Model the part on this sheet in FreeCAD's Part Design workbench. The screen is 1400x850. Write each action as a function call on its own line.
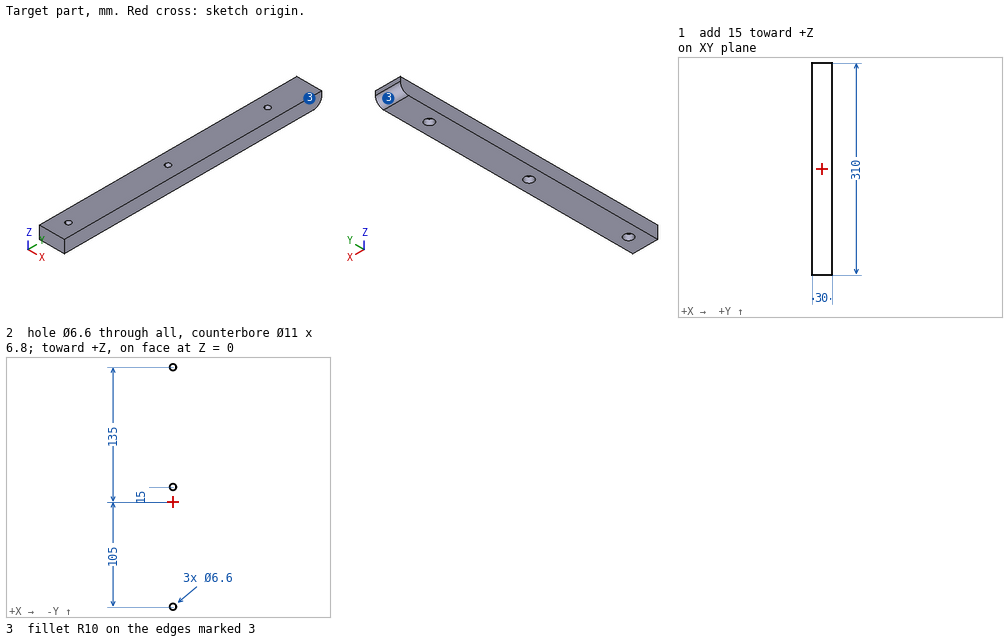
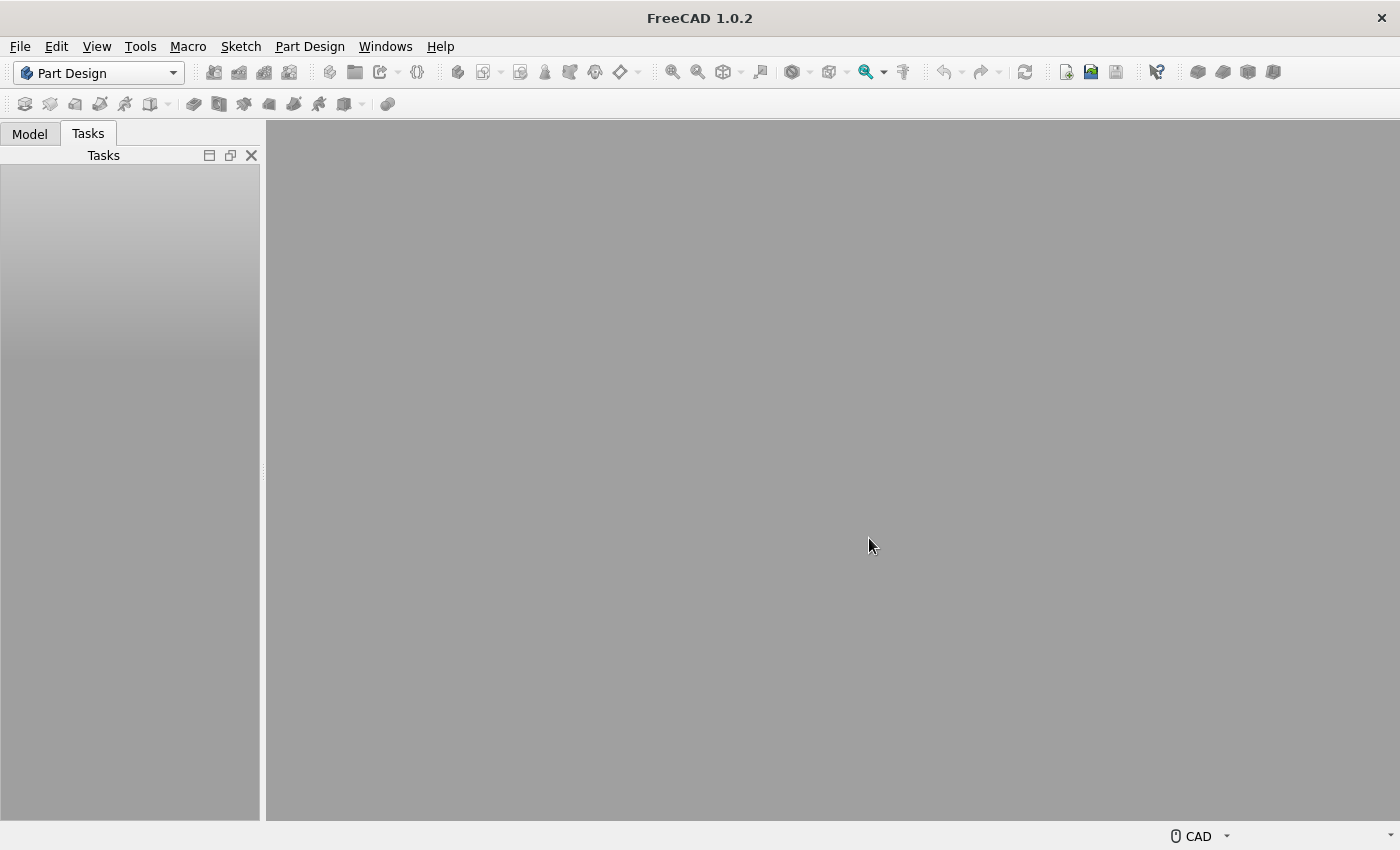
click(1066, 72)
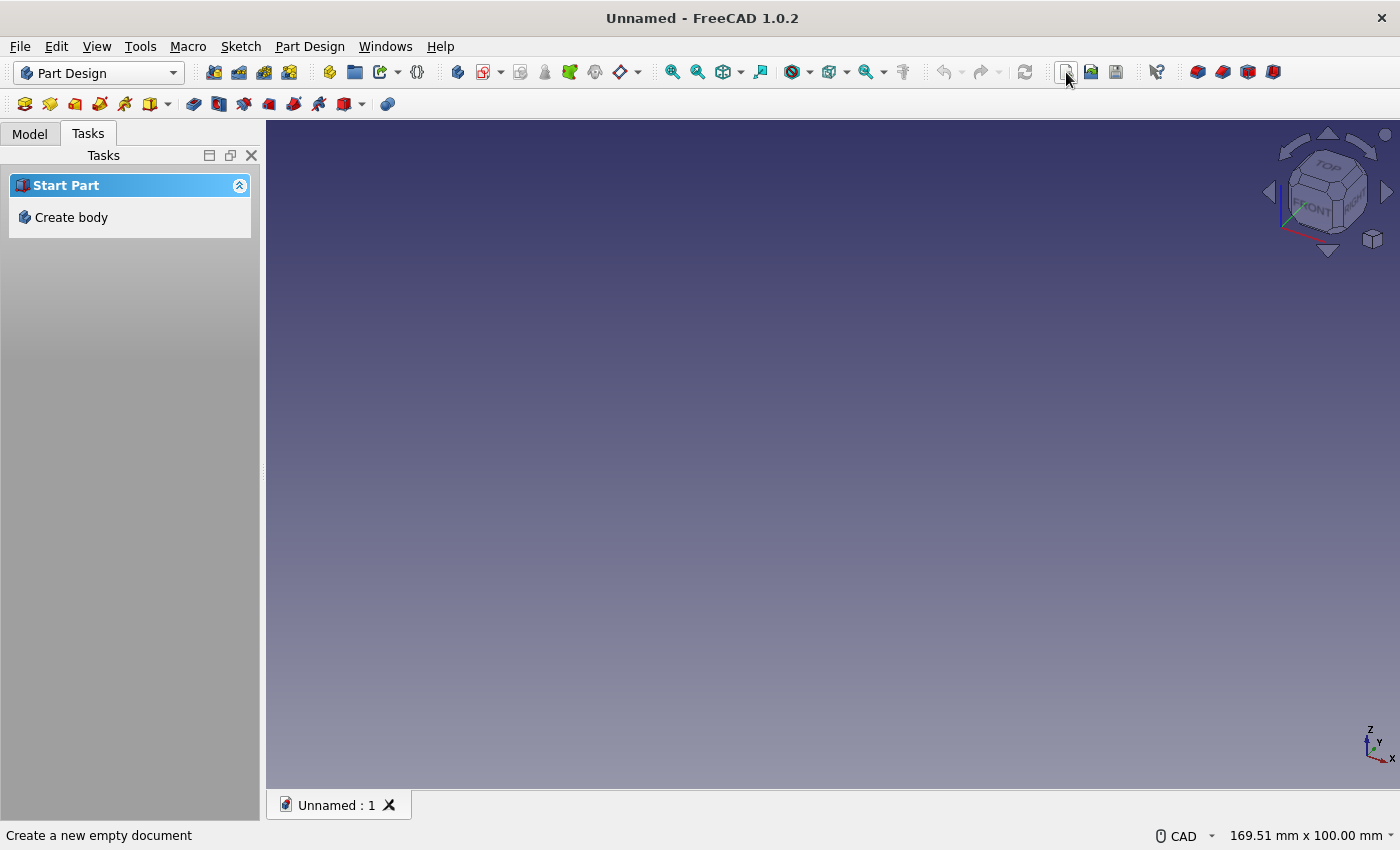
click(482, 72)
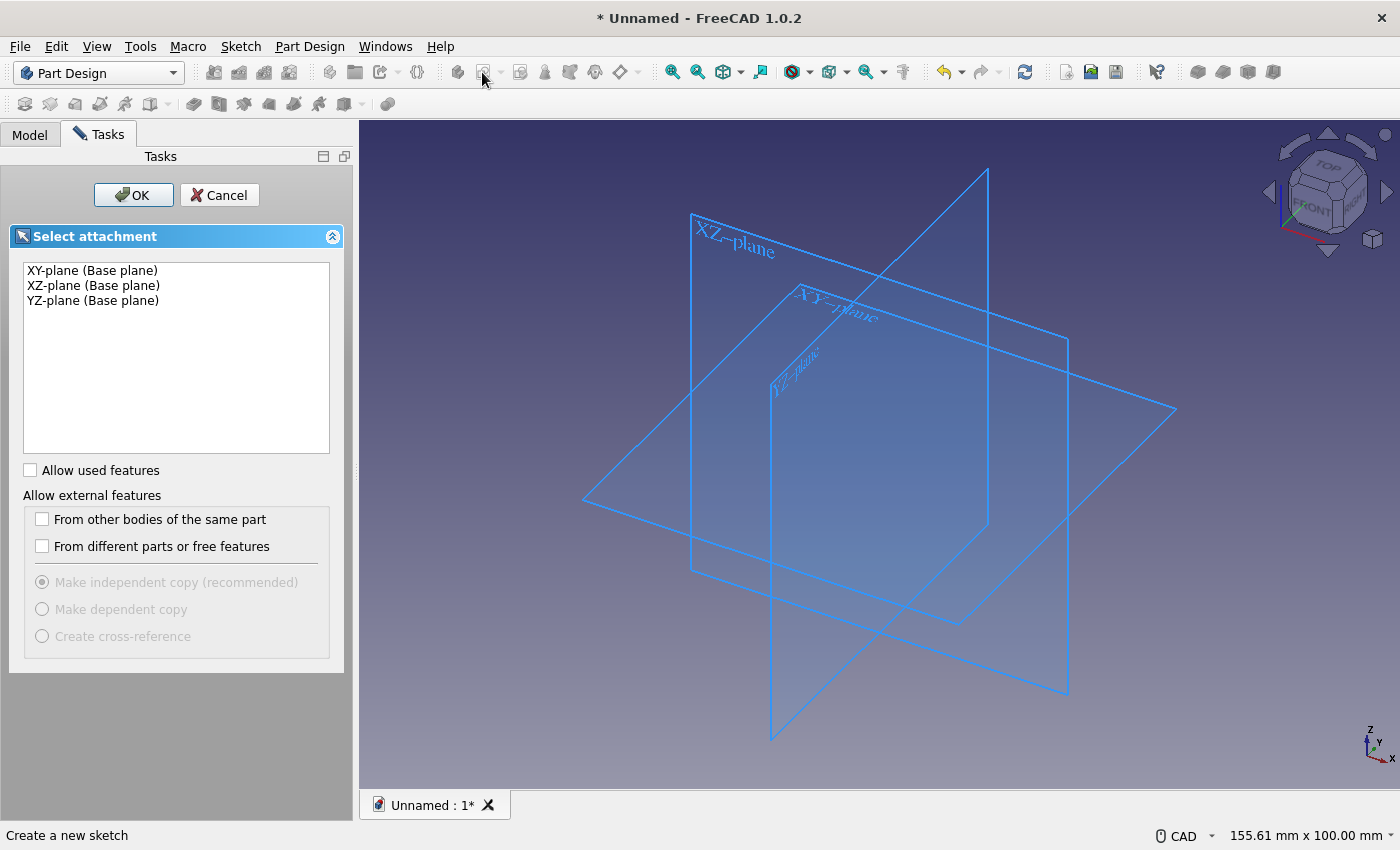
click(84, 270)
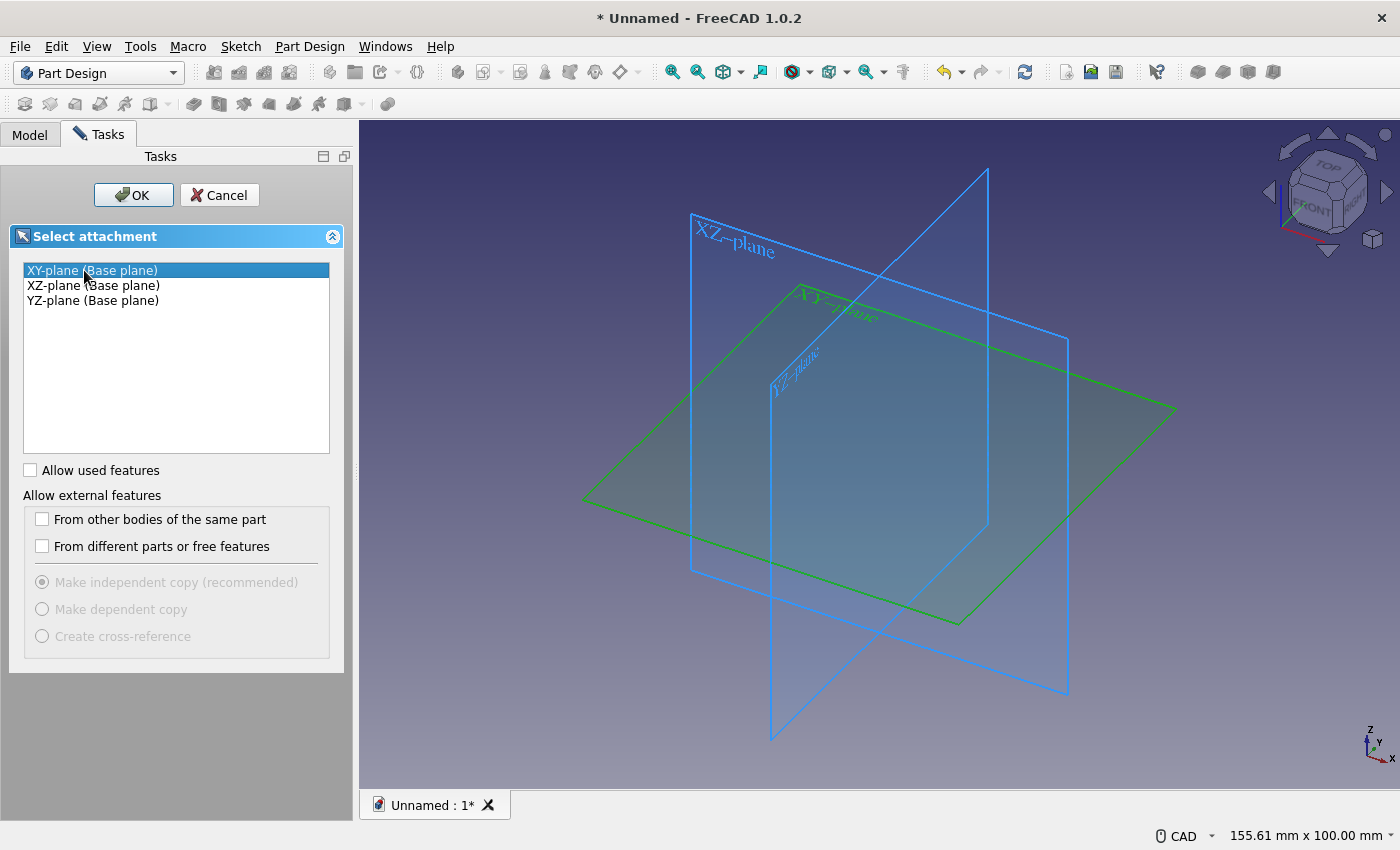
click(134, 195)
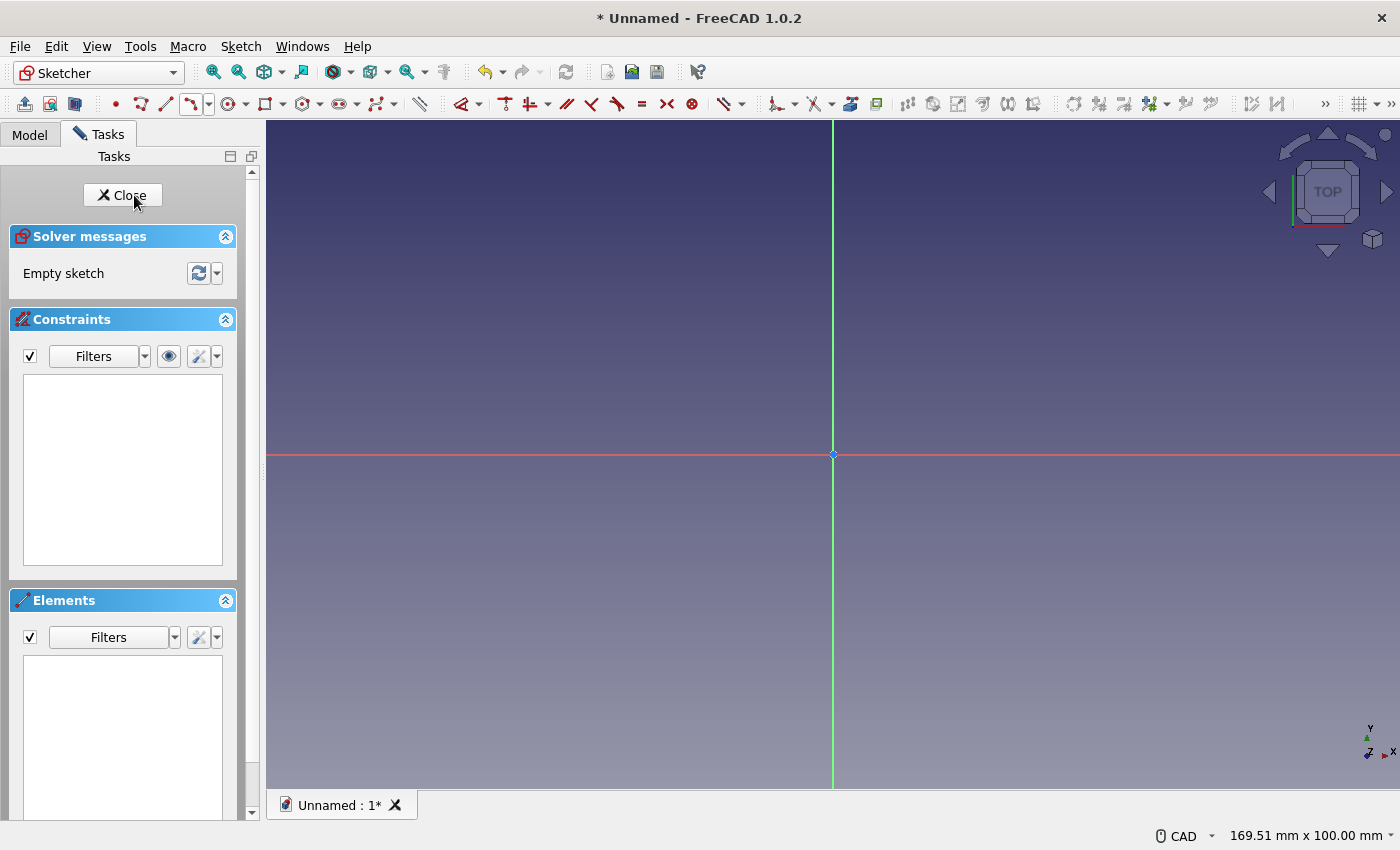
scroll(747, 454, down, 8)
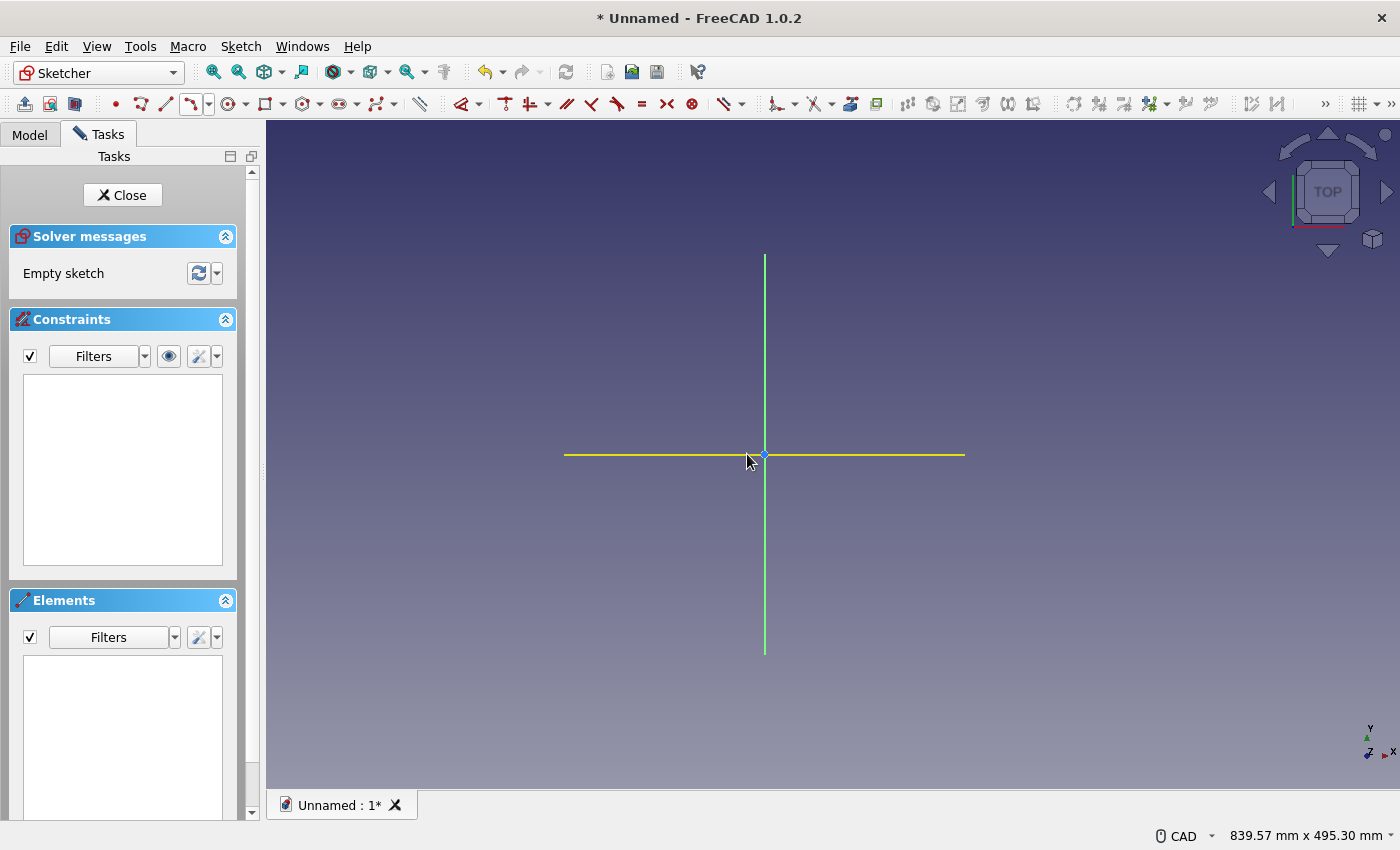
key(g)
key(v)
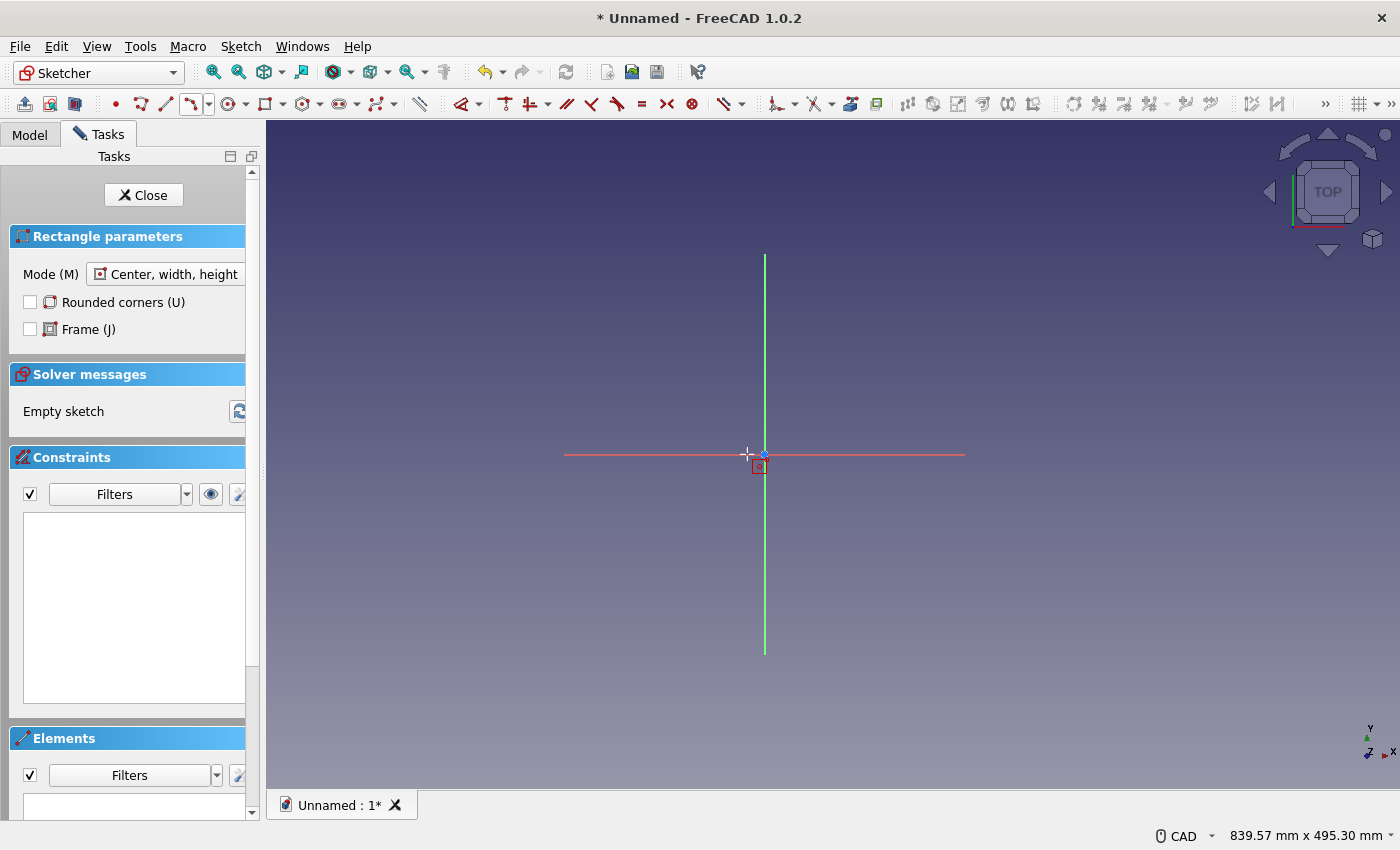
click(765, 454)
click(785, 245)
key(Escape)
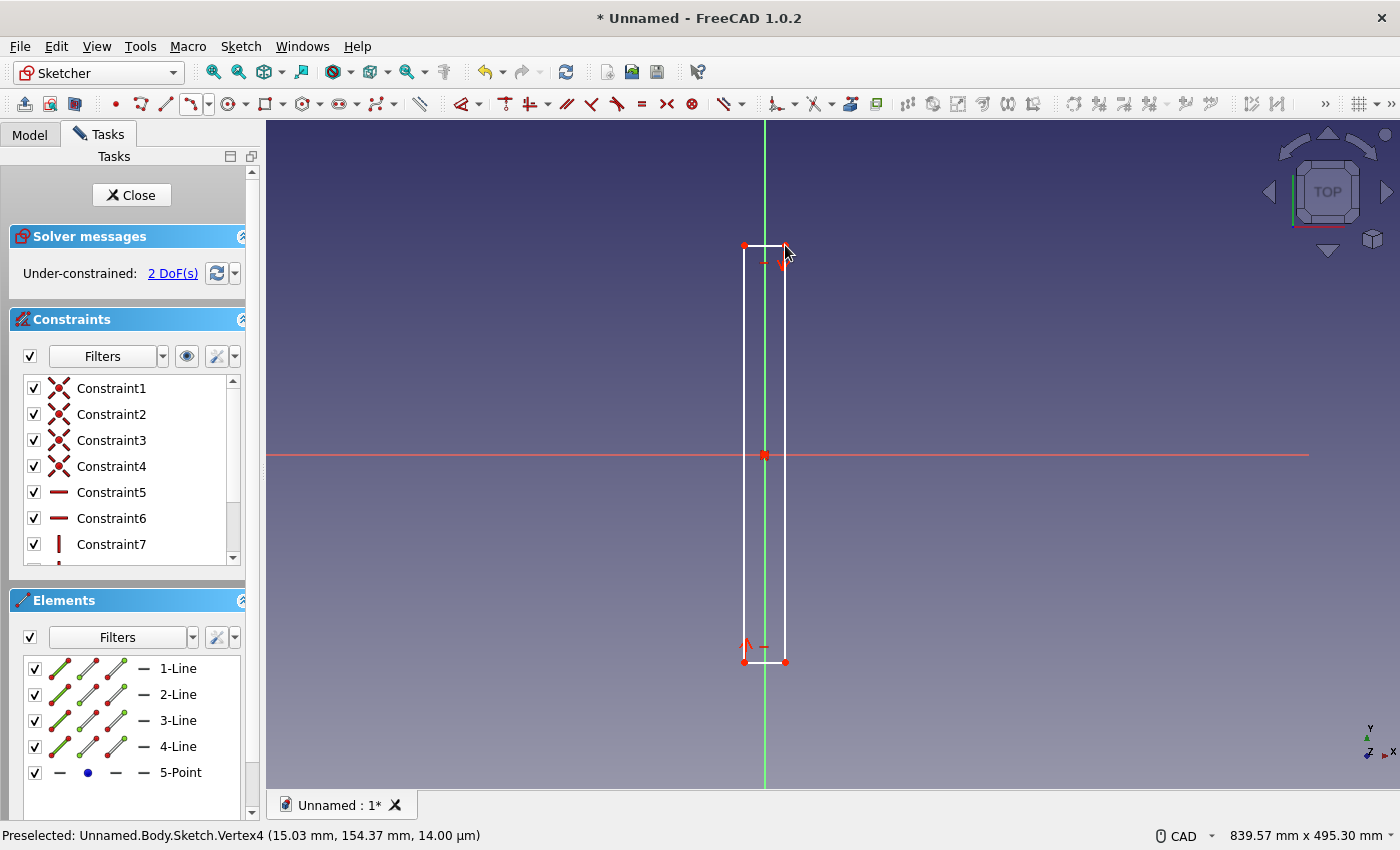
click(460, 104)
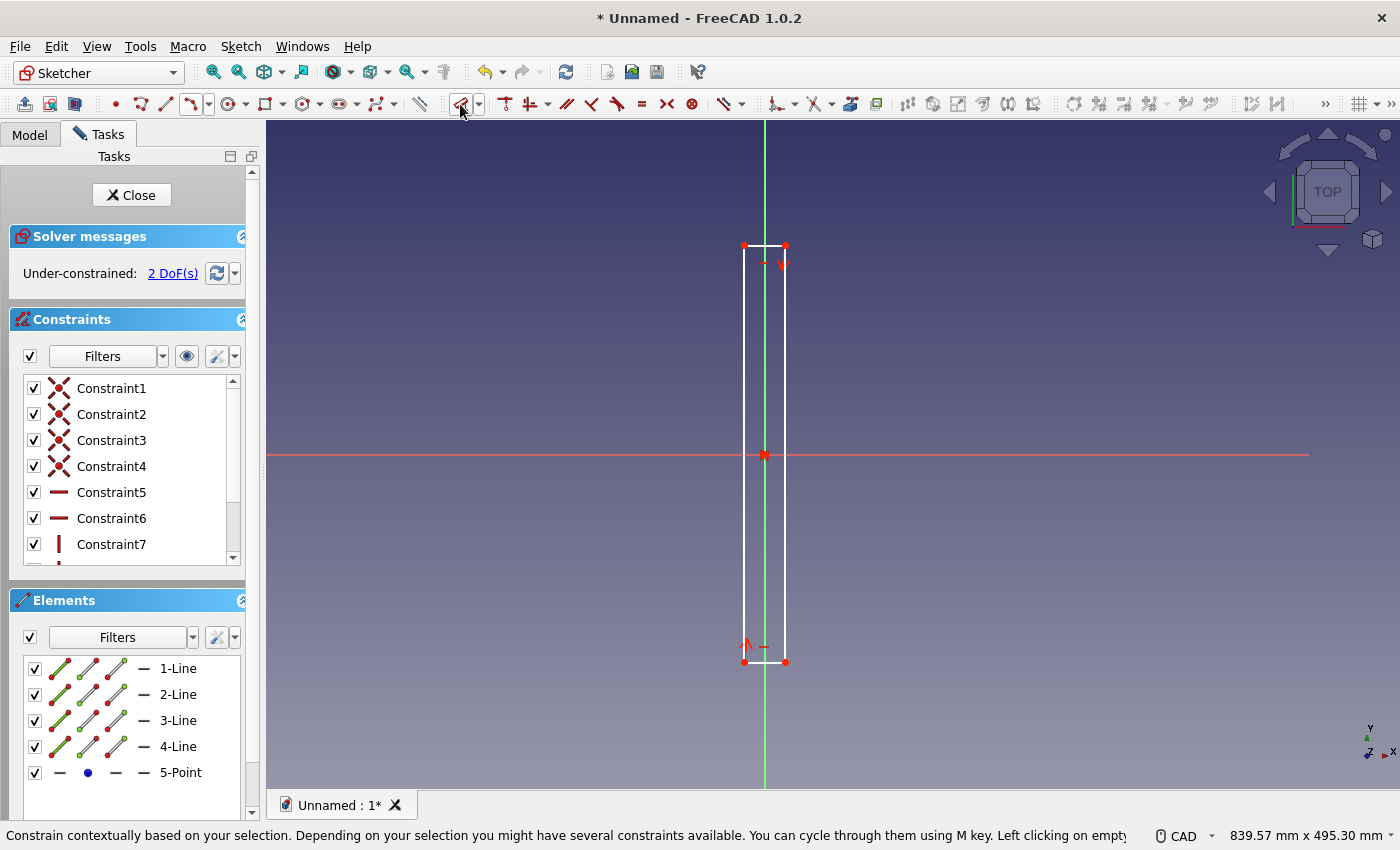
click(765, 663)
click(750, 697)